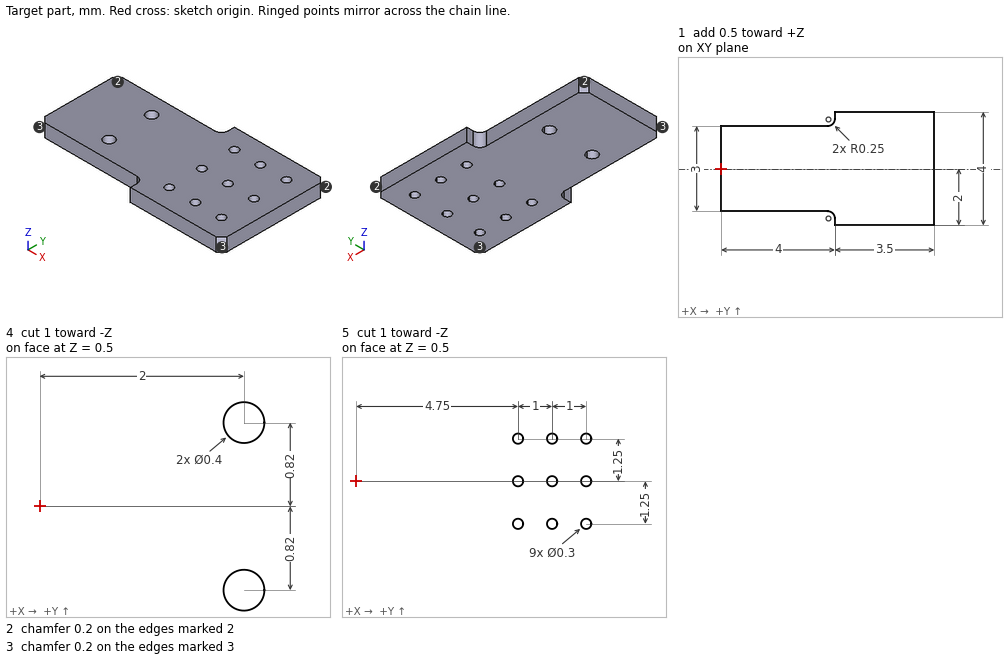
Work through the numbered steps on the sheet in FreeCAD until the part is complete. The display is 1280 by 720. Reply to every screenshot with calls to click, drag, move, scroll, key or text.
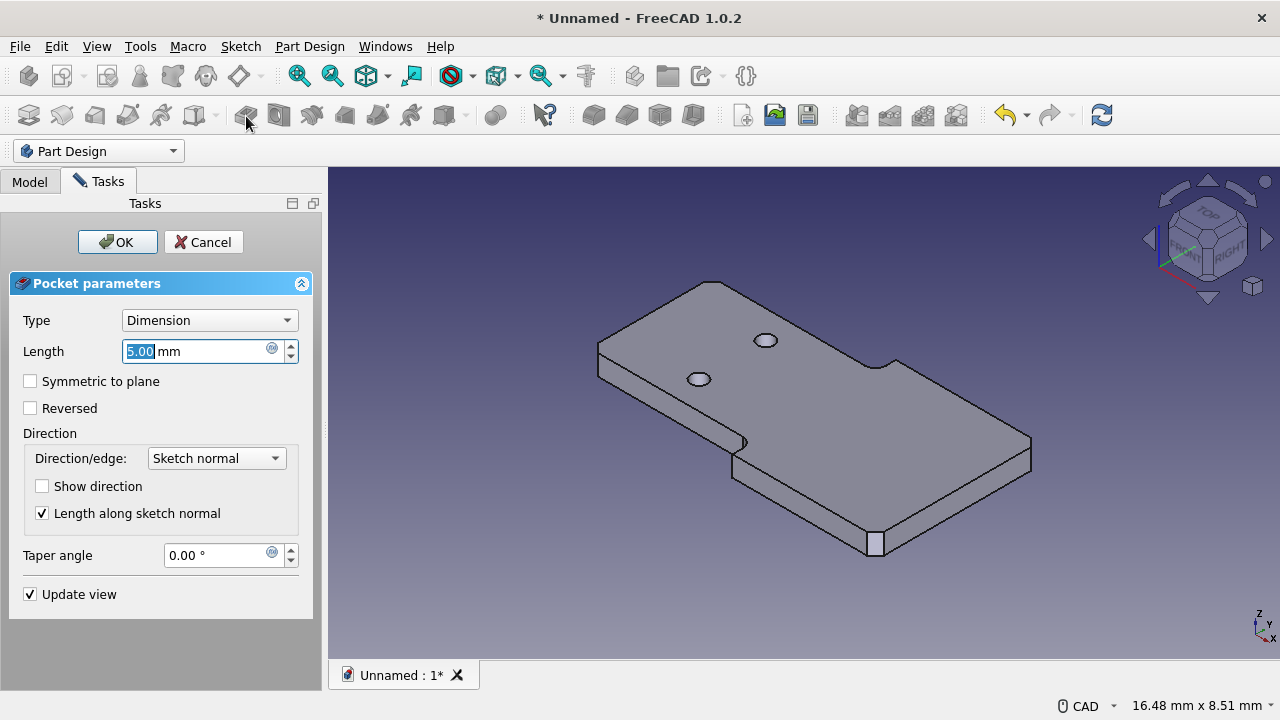
text(1)
key(Tab)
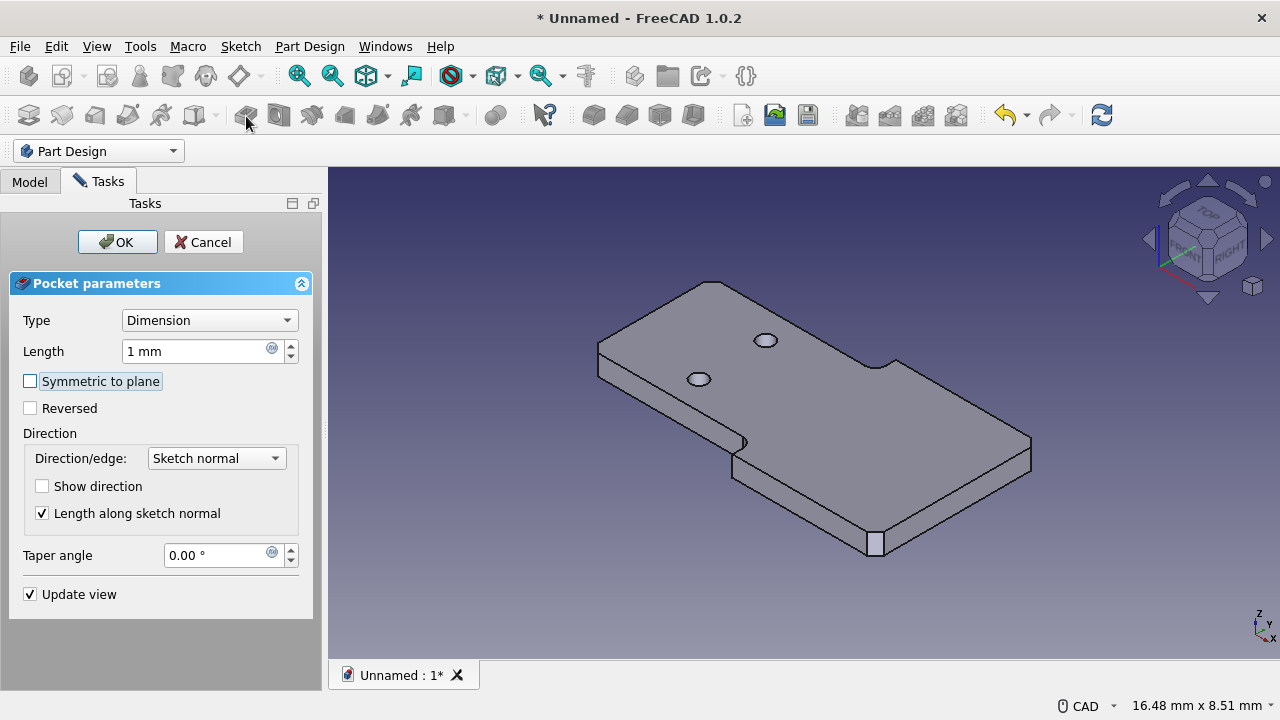
click(118, 242)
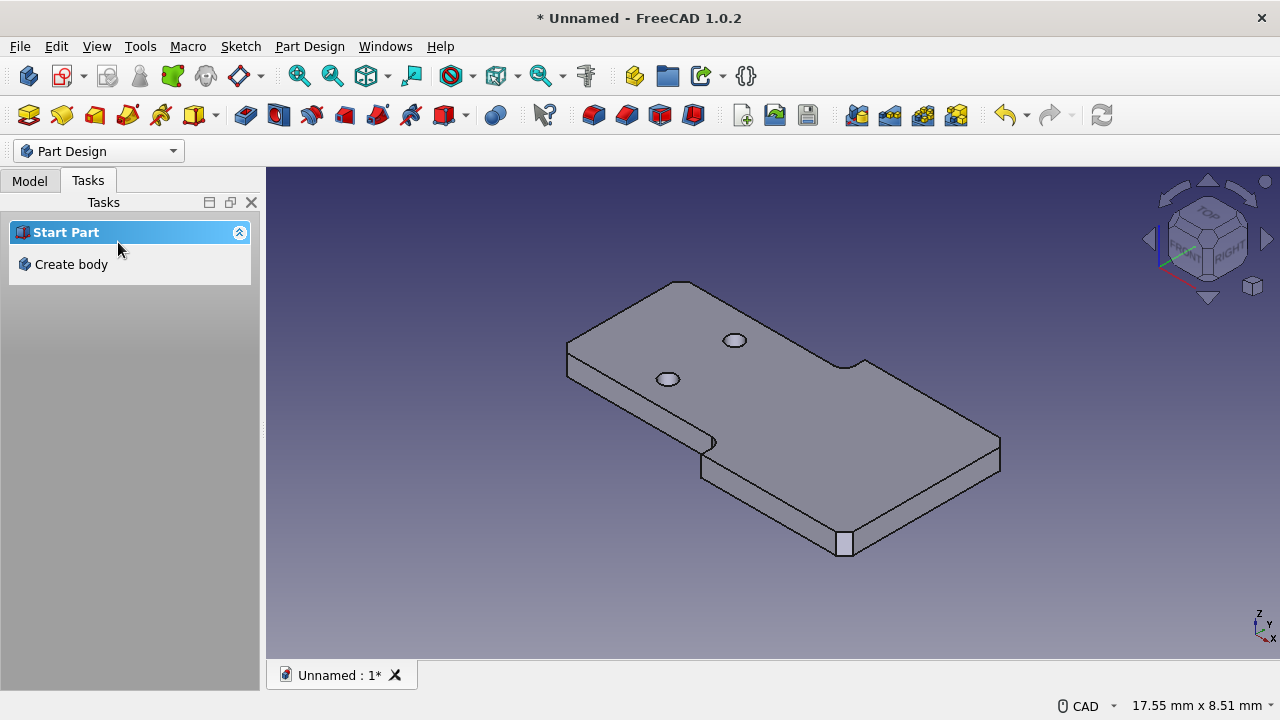
click(817, 425)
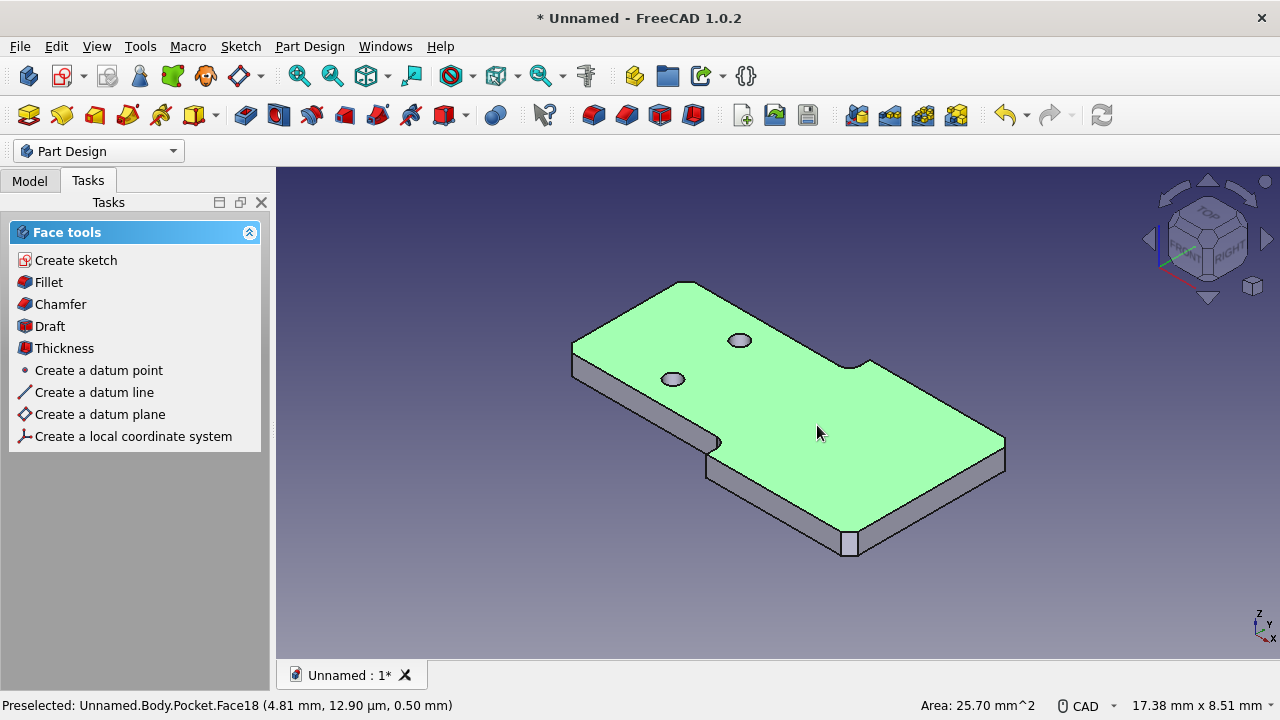
click(62, 76)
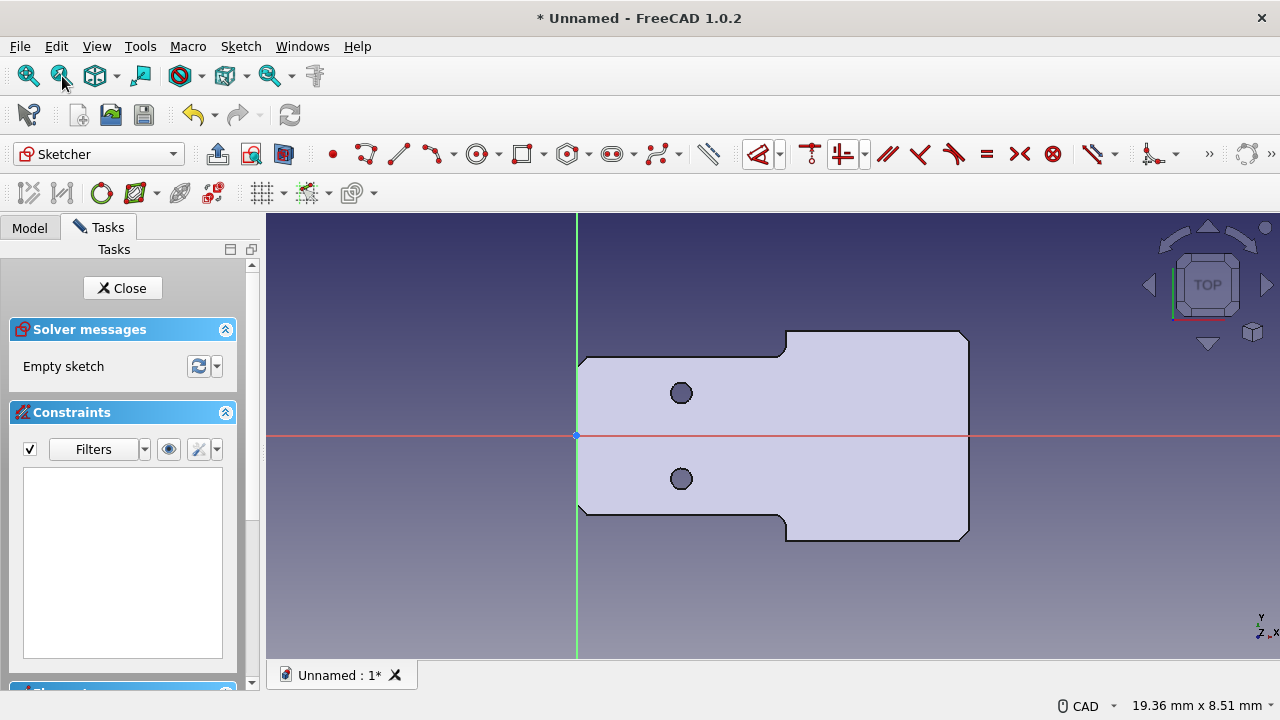
scroll(865, 436, up, 2)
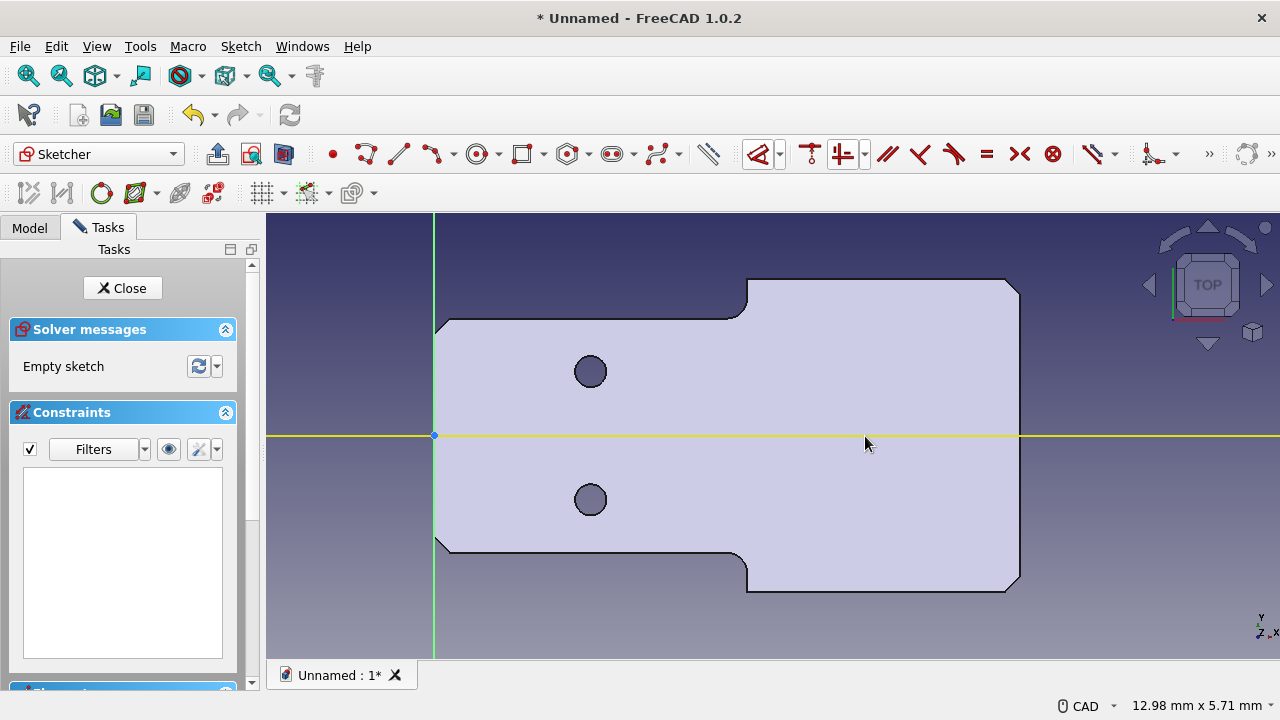
key(g)
key(c)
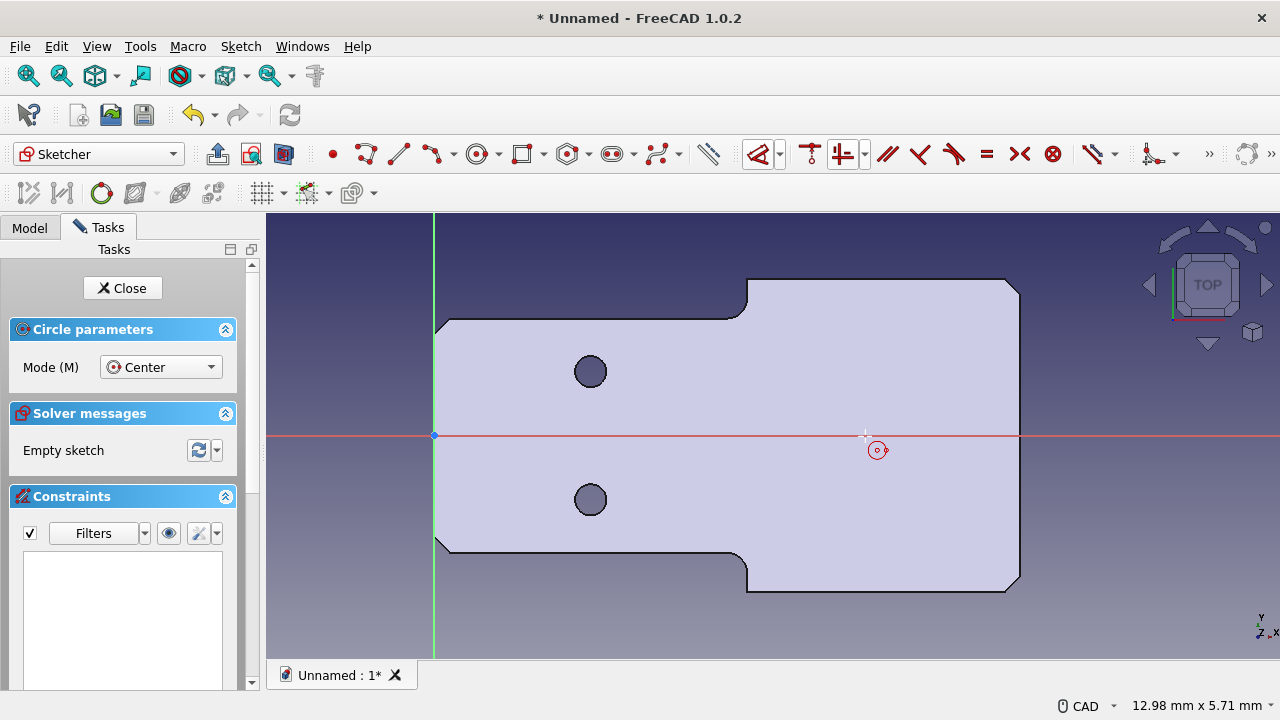
scroll(806, 338, up, 4)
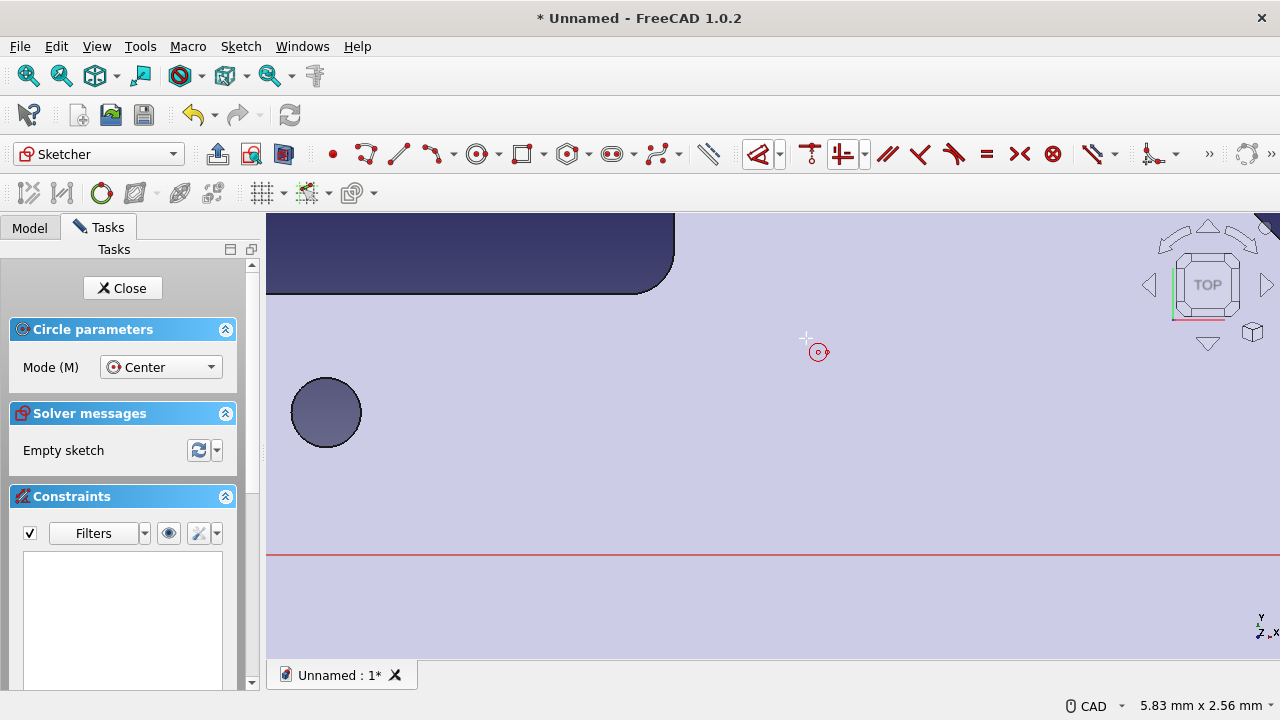
click(804, 338)
click(823, 319)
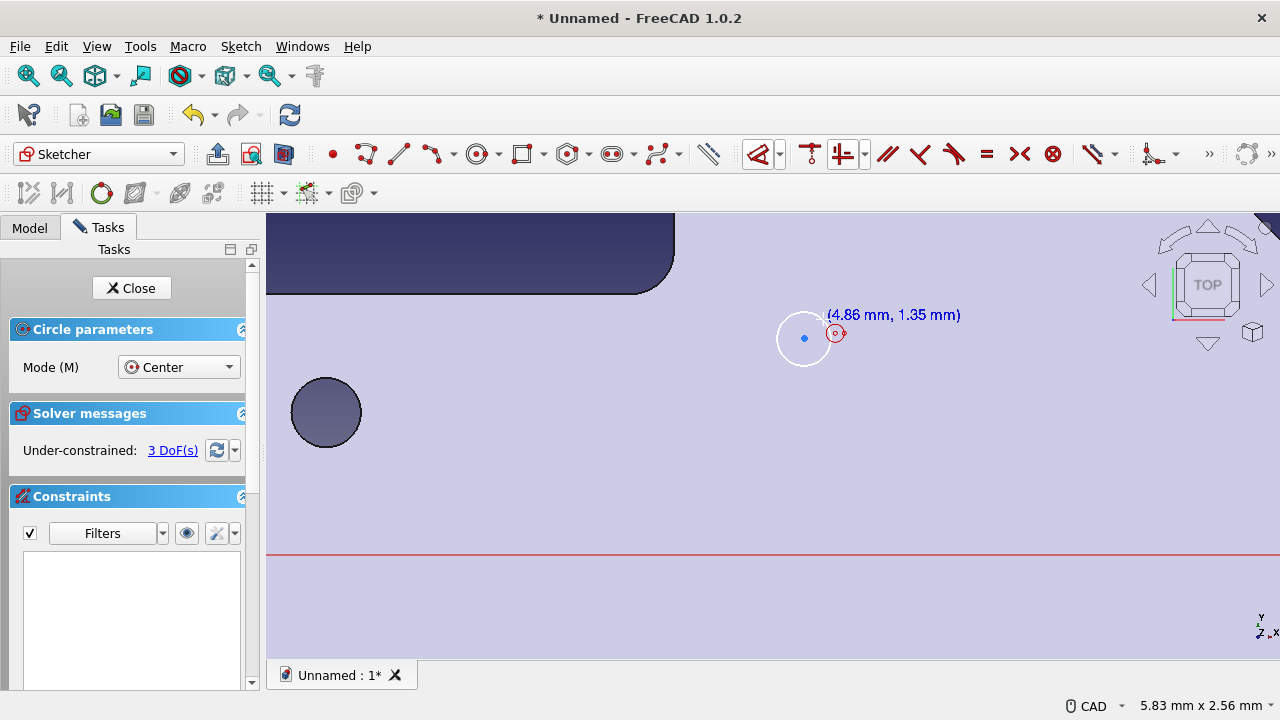
click(978, 338)
click(997, 319)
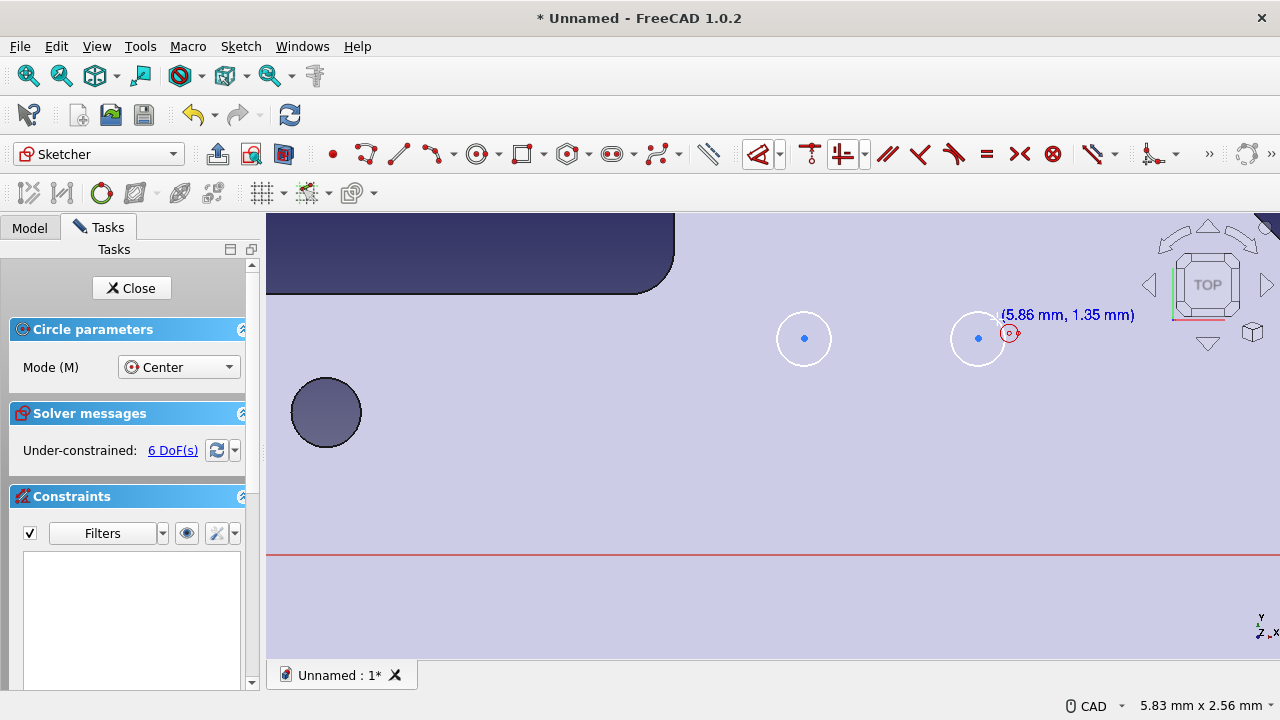
scroll(807, 339, down, 4)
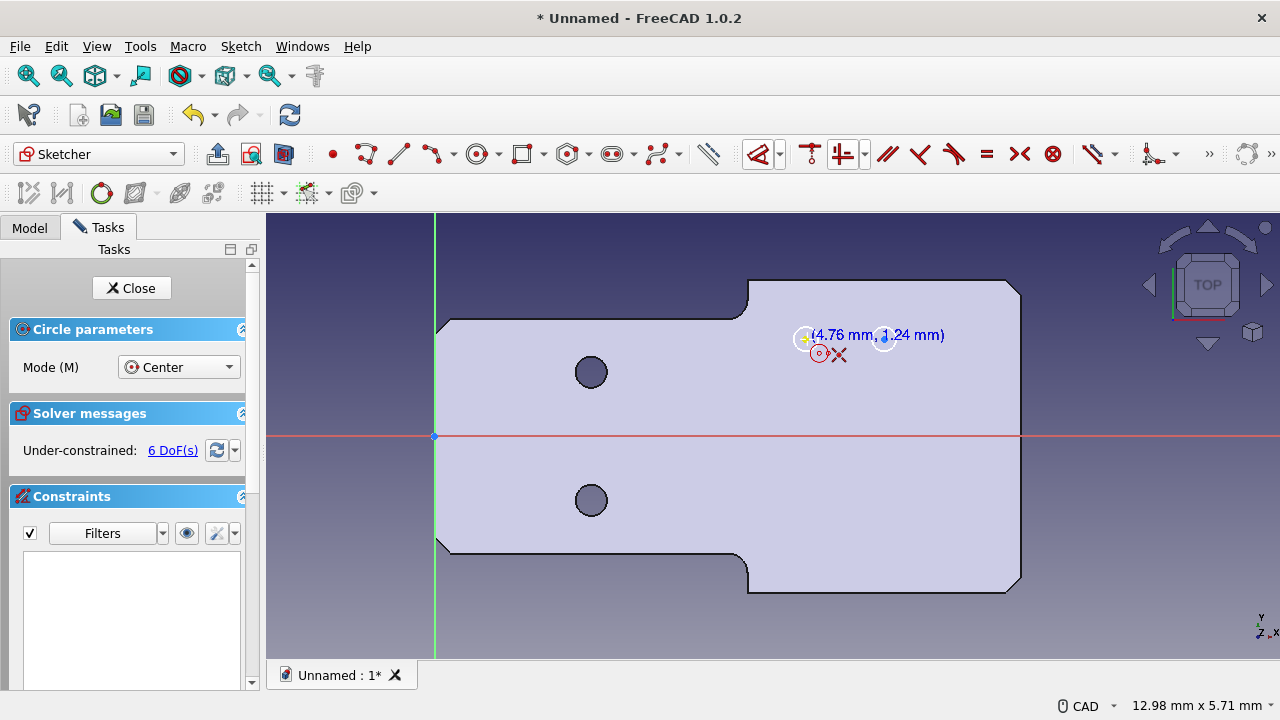
scroll(962, 339, up, 4)